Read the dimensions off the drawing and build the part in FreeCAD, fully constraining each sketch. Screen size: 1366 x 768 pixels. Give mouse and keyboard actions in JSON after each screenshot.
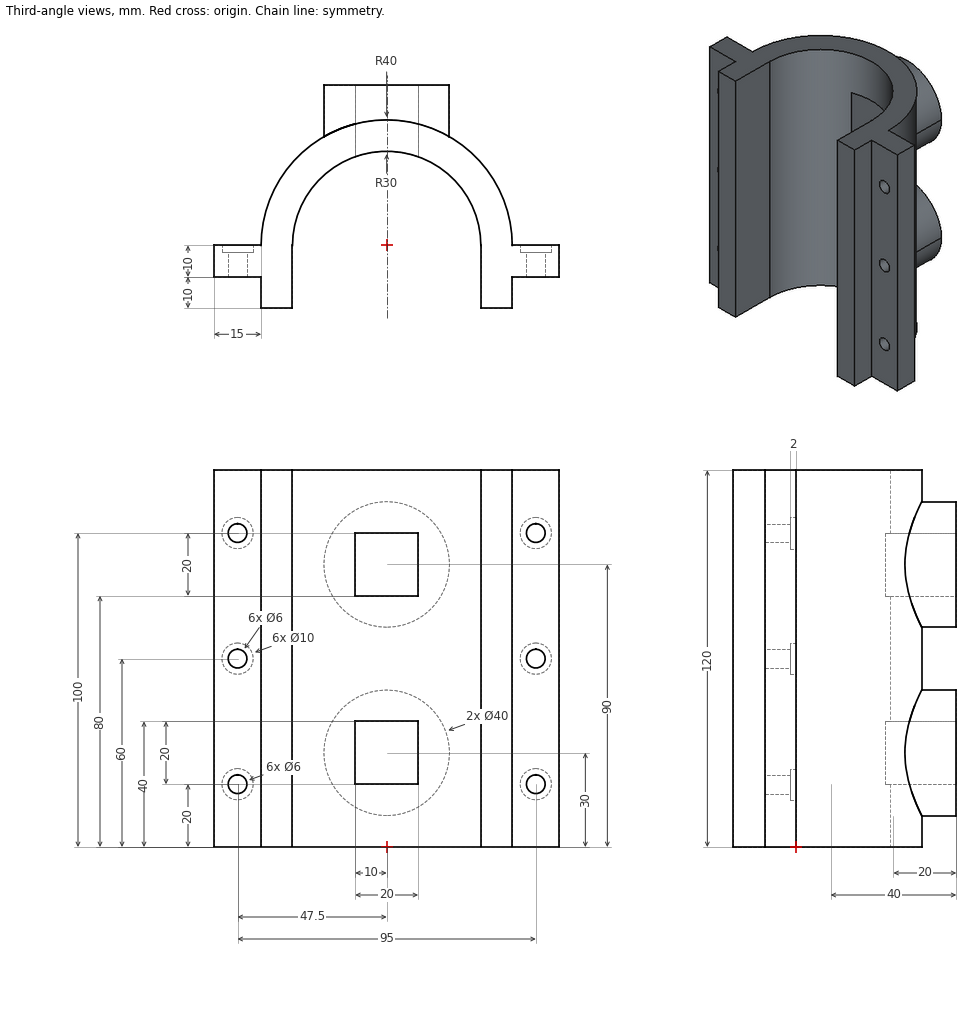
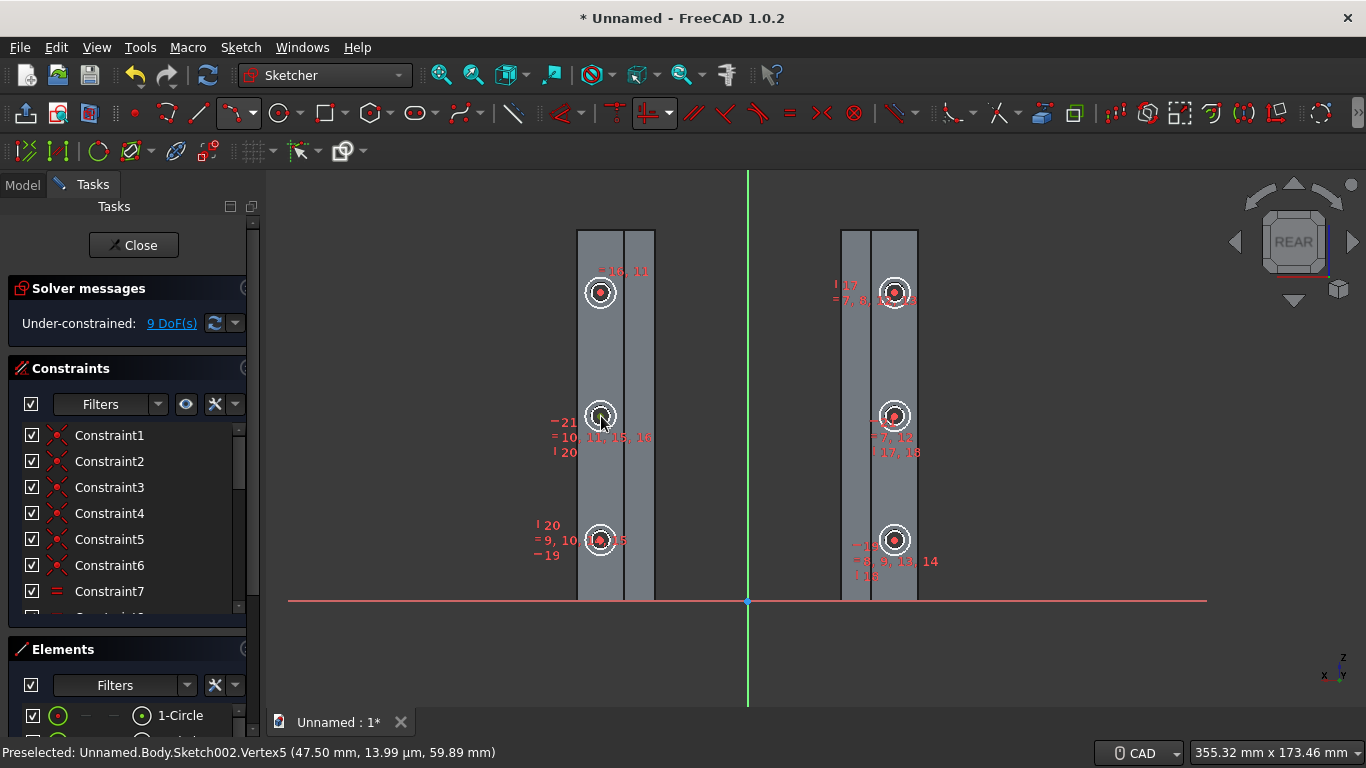
{"action": "left_click", "coordinate": [601, 293]}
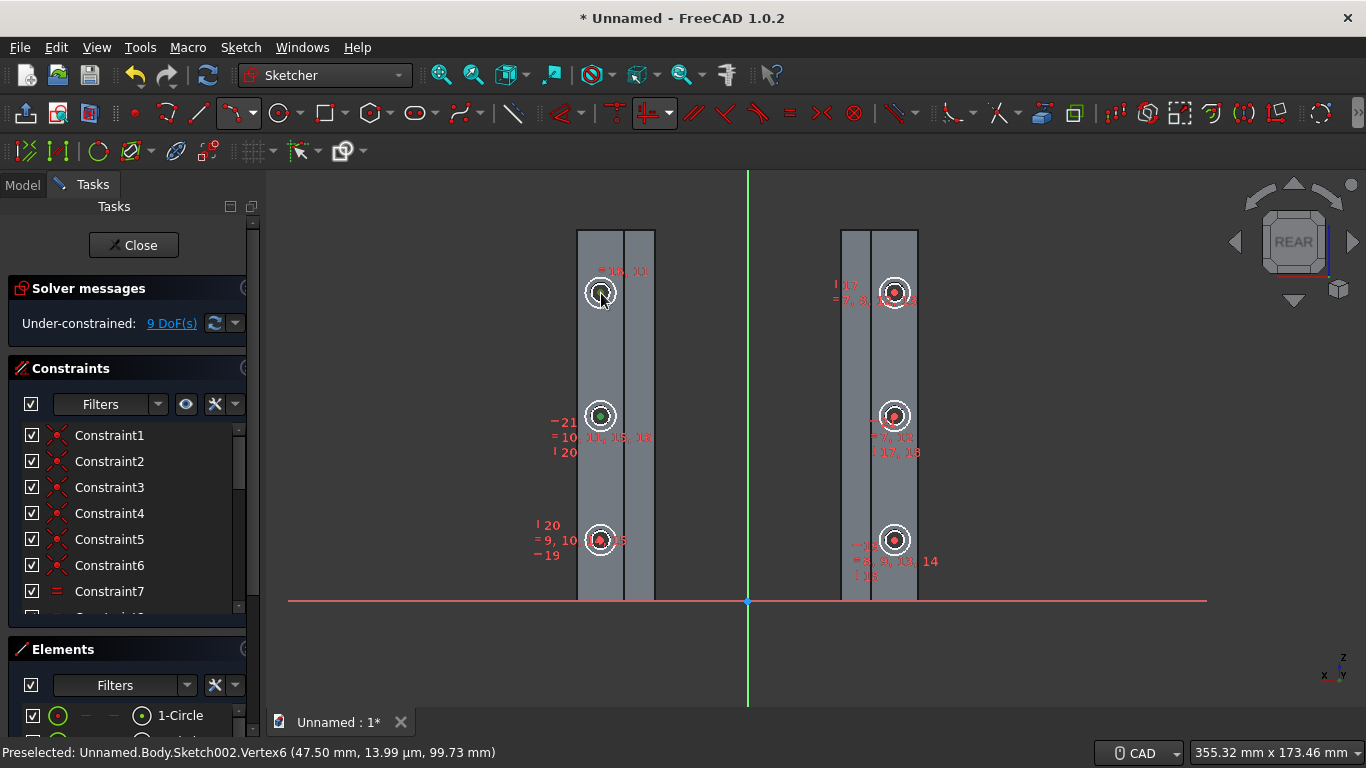
{"action": "left_click", "coordinate": [672, 114]}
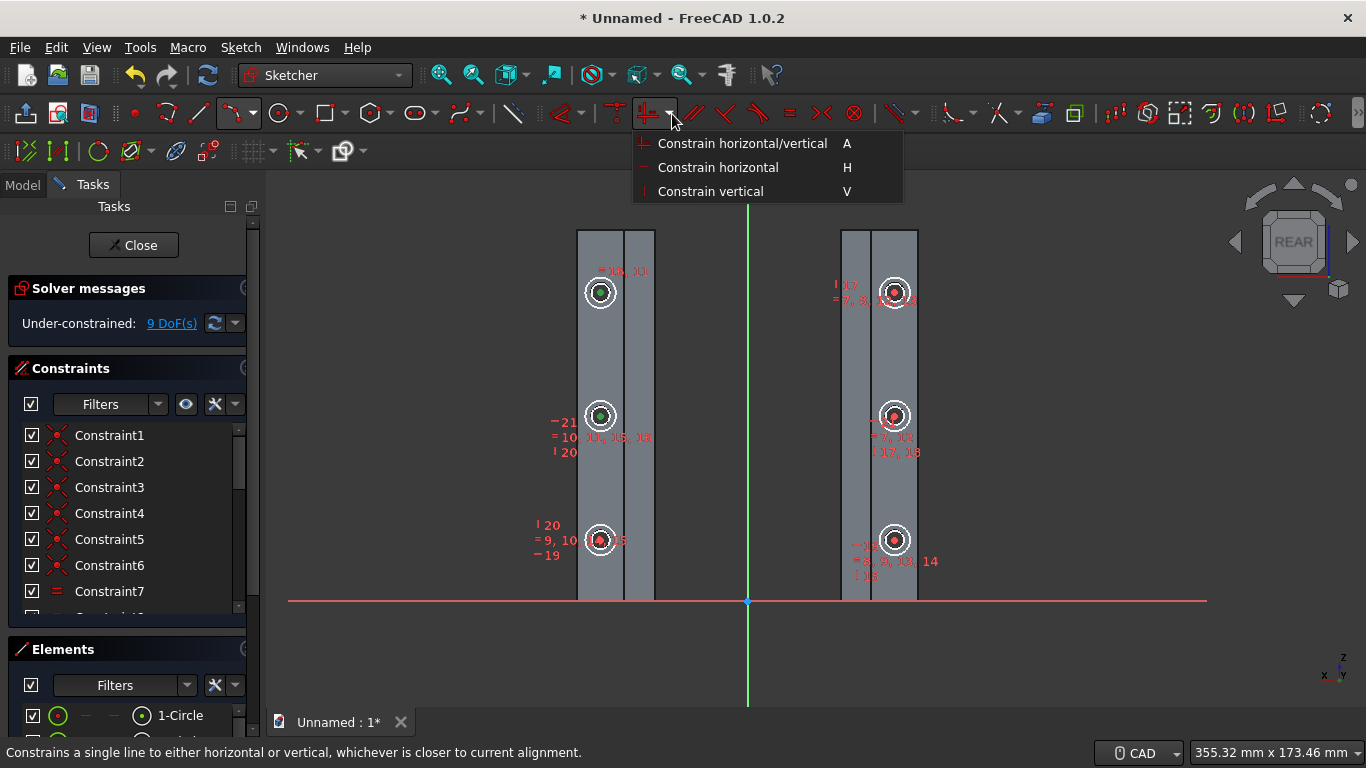
{"action": "left_click", "coordinate": [768, 191]}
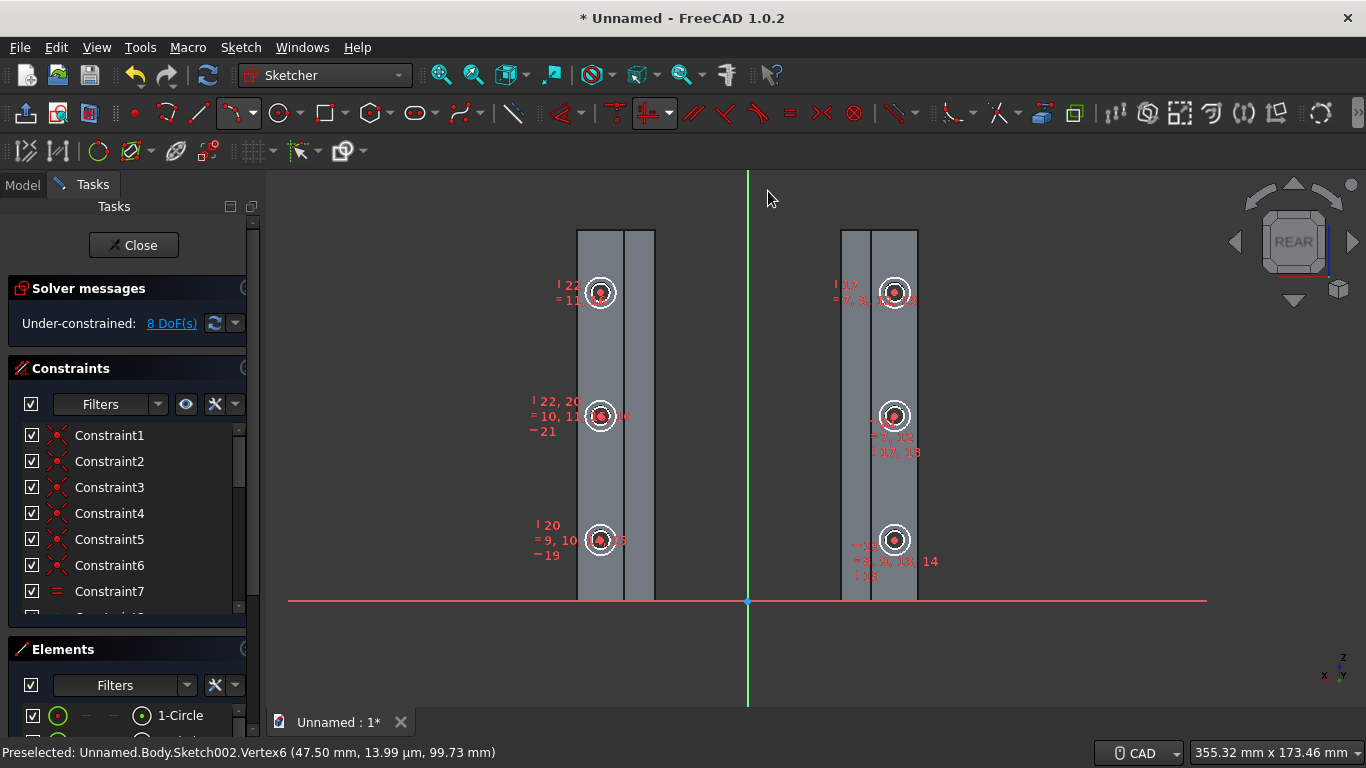
{"action": "scroll", "coordinate": [895, 293], "scroll_direction": "up", "scroll_amount": 4}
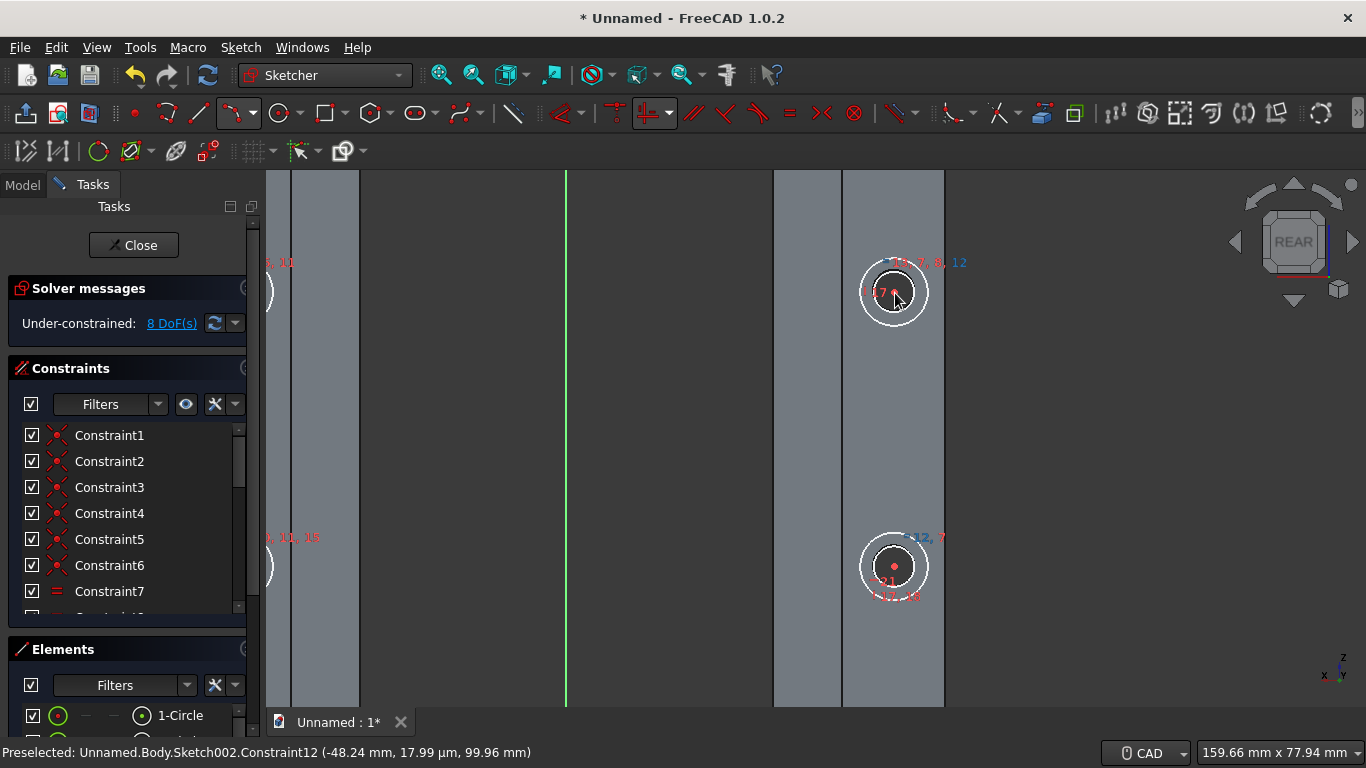
{"action": "left_click", "coordinate": [894, 292]}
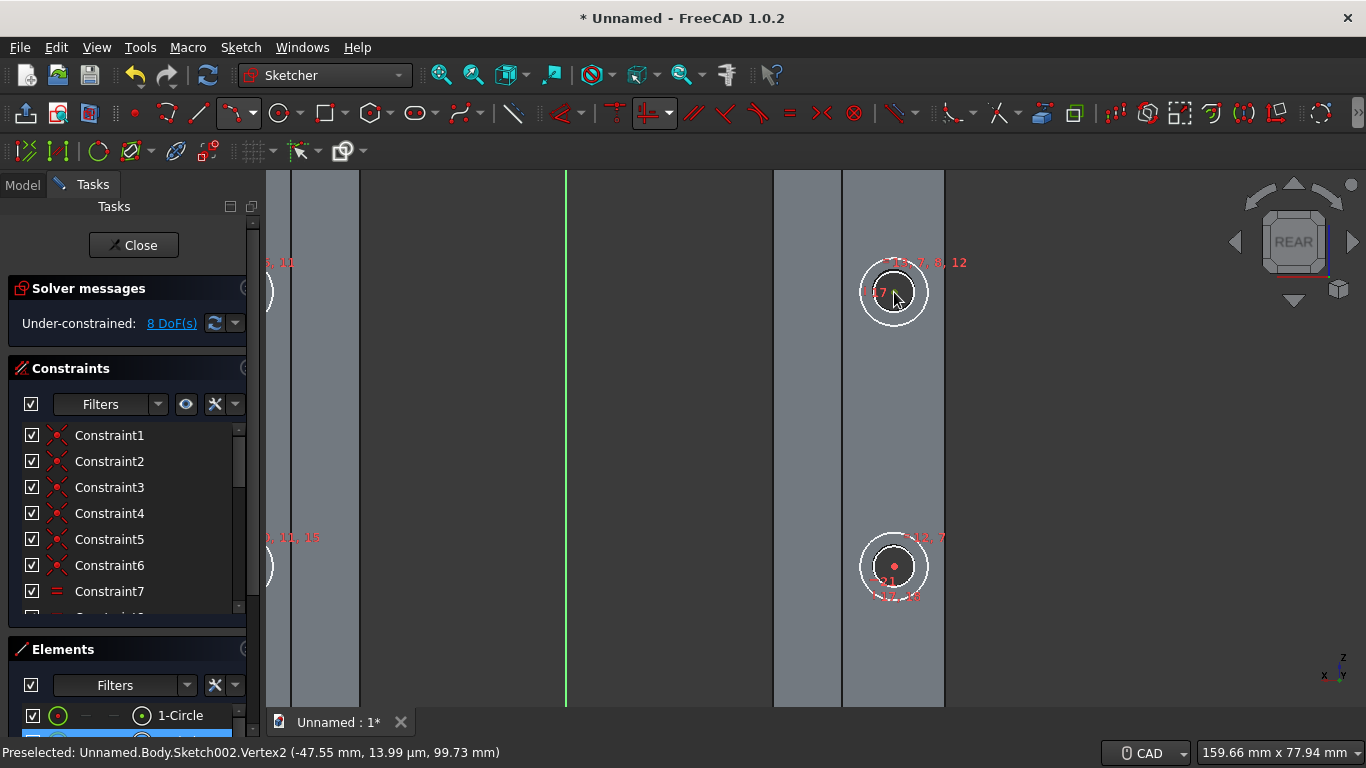
{"action": "scroll", "coordinate": [895, 292], "scroll_direction": "down", "scroll_amount": 4}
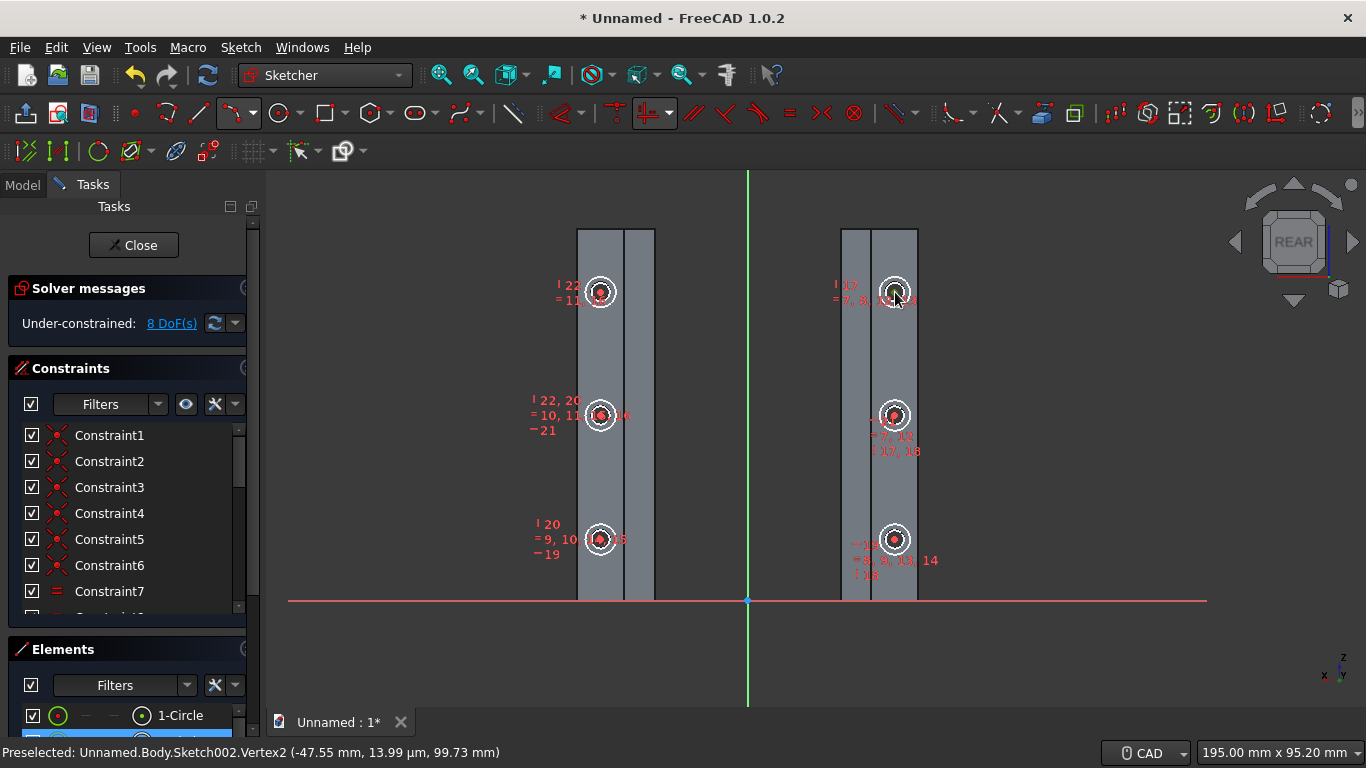
{"action": "scroll", "coordinate": [601, 292], "scroll_direction": "up", "scroll_amount": 4}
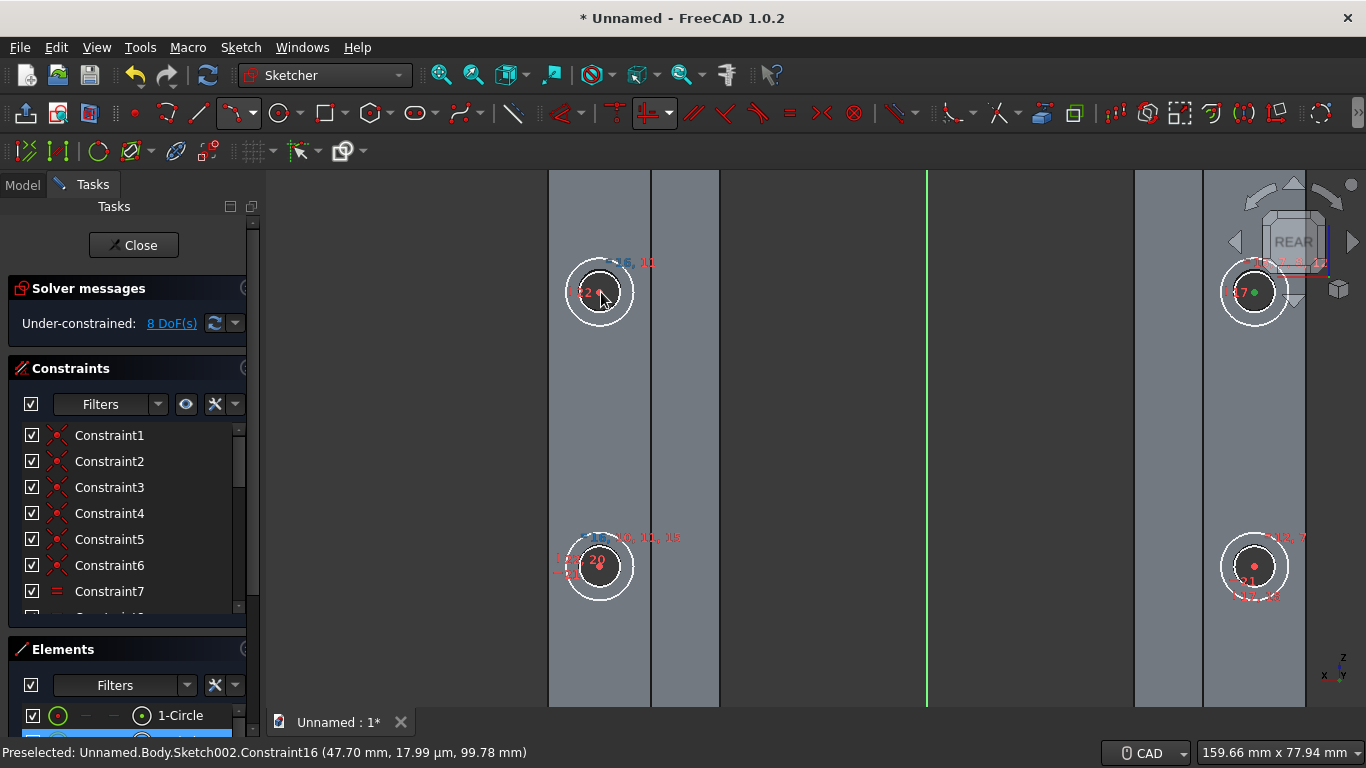
{"action": "left_click", "coordinate": [600, 292]}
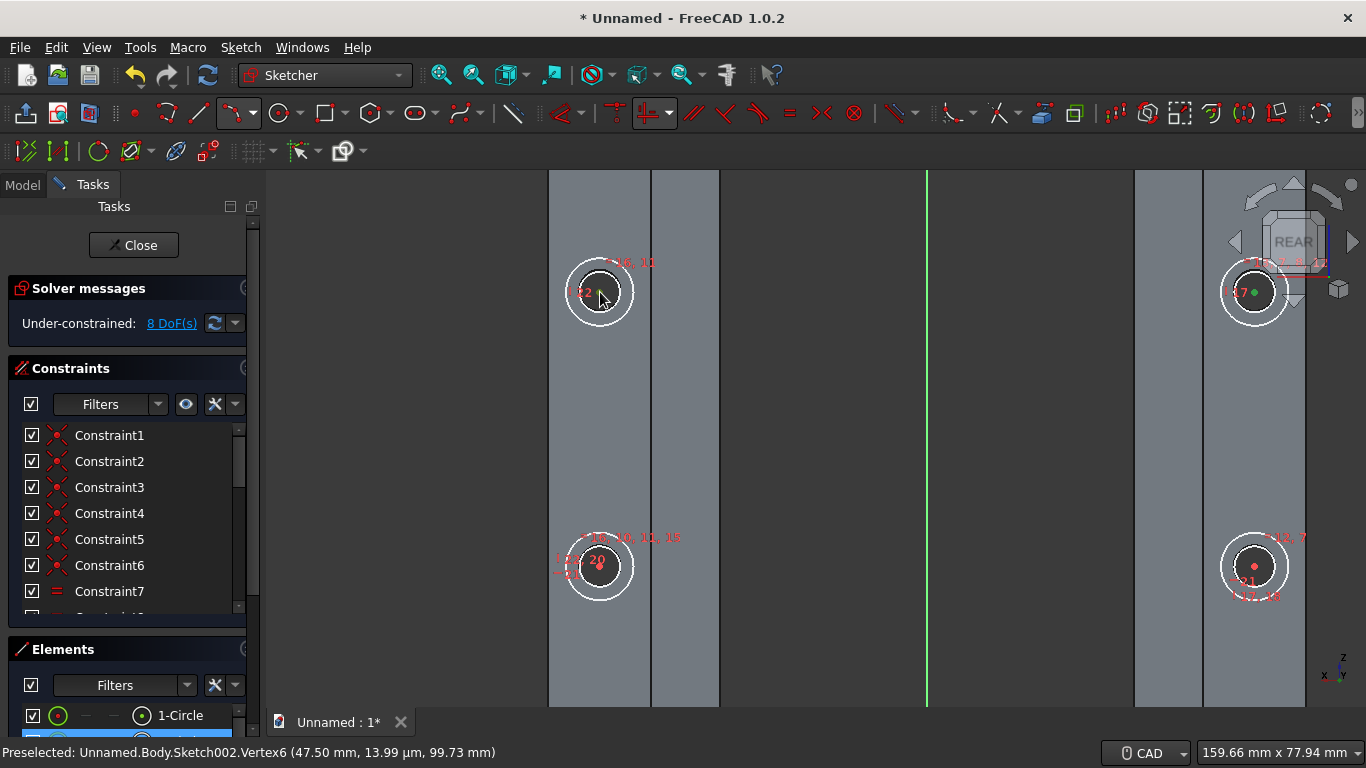
{"action": "left_click", "coordinate": [672, 114]}